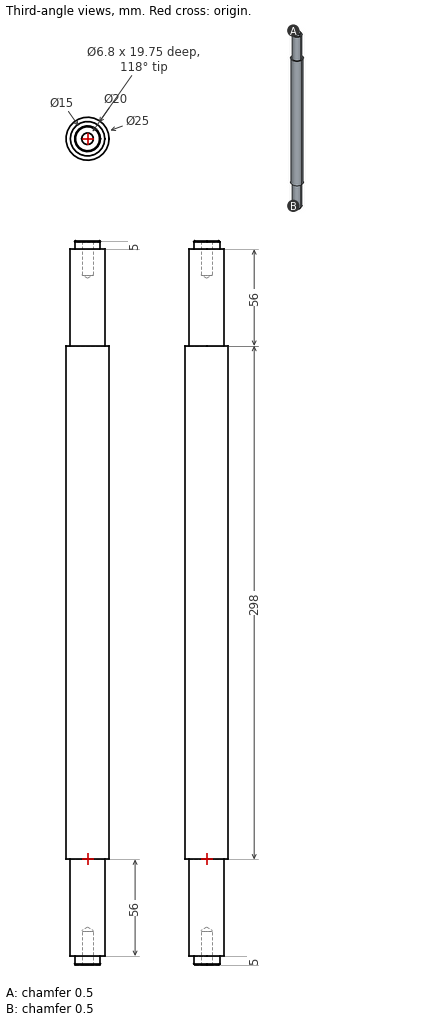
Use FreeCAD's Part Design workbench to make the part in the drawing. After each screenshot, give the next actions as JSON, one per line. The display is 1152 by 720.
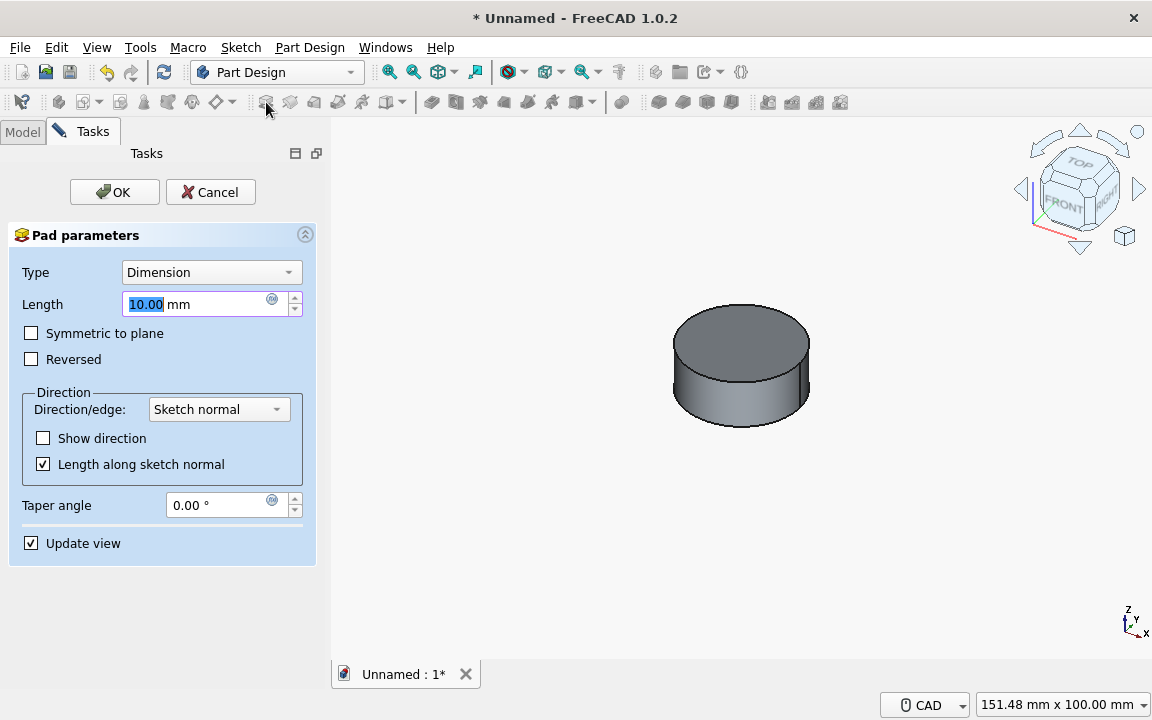
{"action": "type", "text": "298"}
{"action": "key", "text": "Tab"}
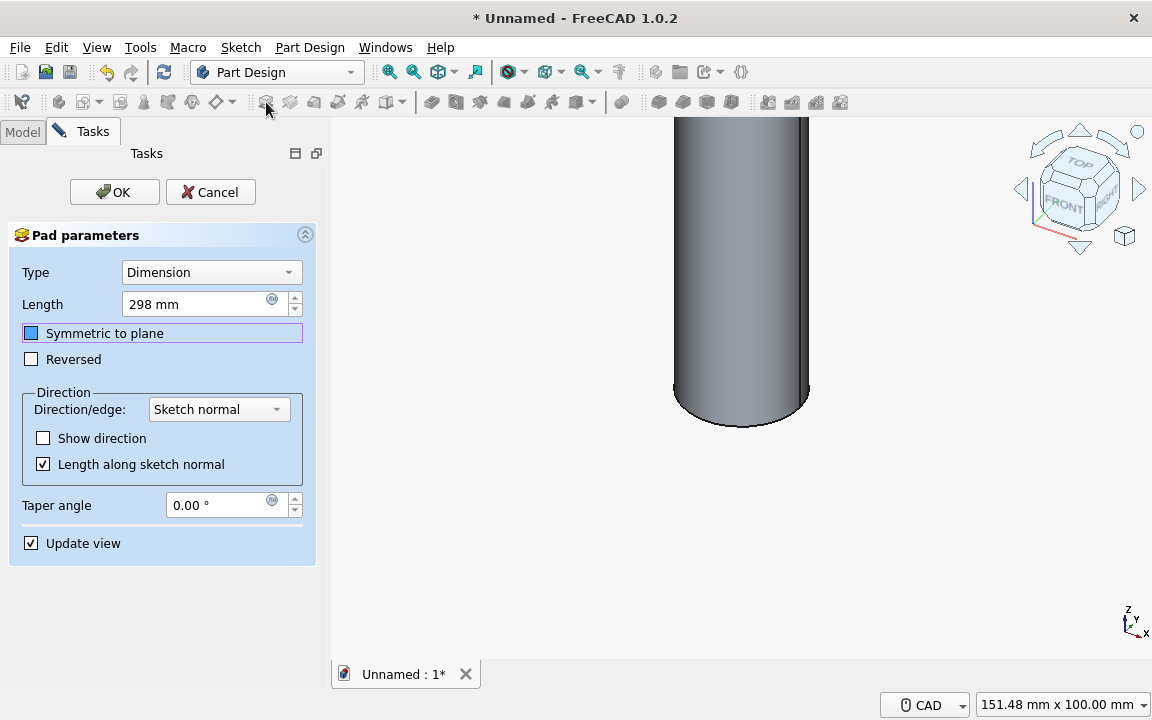
{"action": "left_click", "coordinate": [115, 192]}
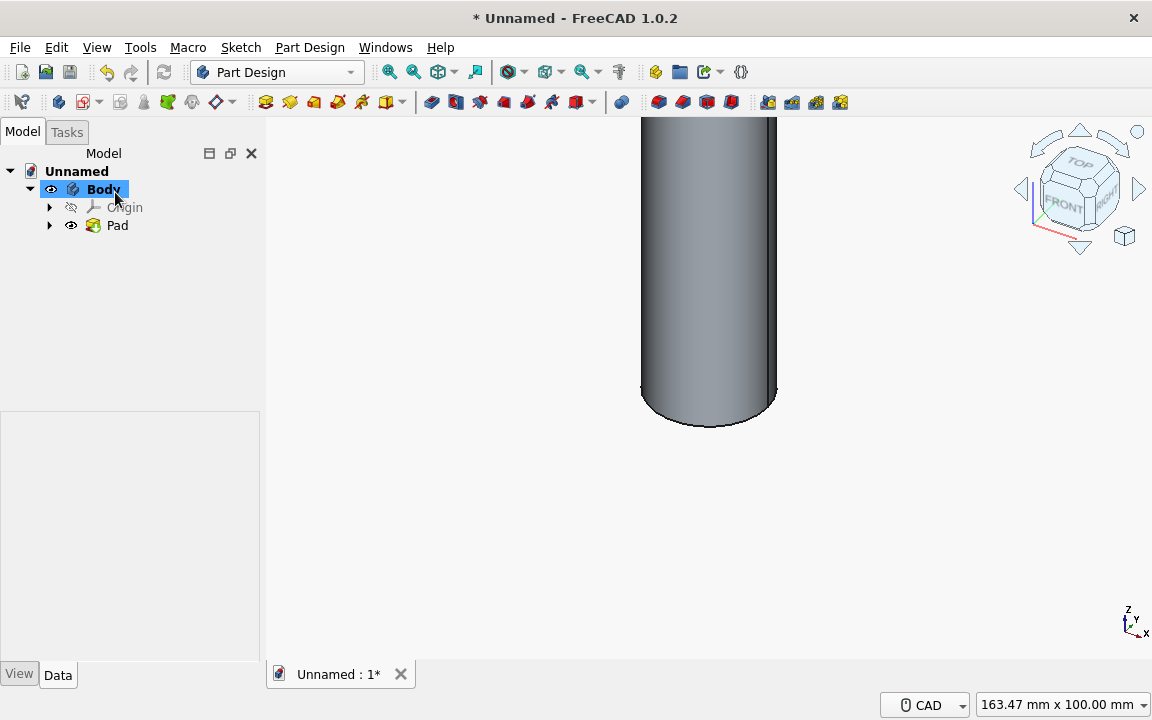
{"action": "left_click", "coordinate": [390, 72]}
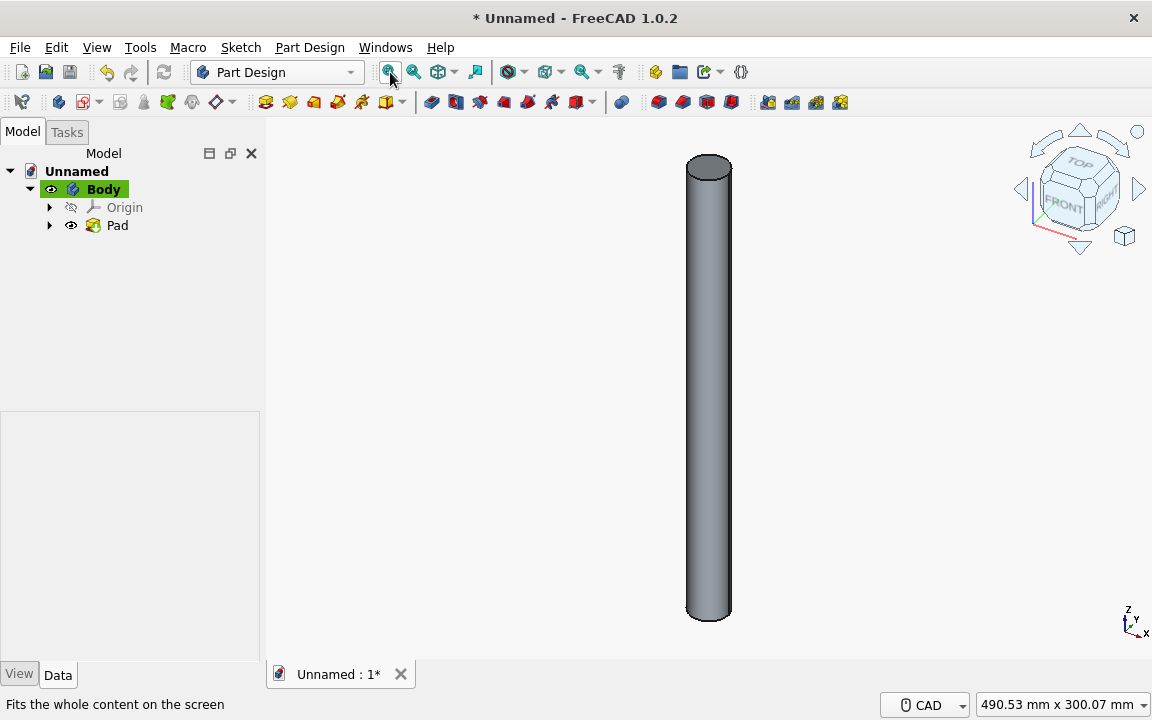
{"action": "key", "text": "5"}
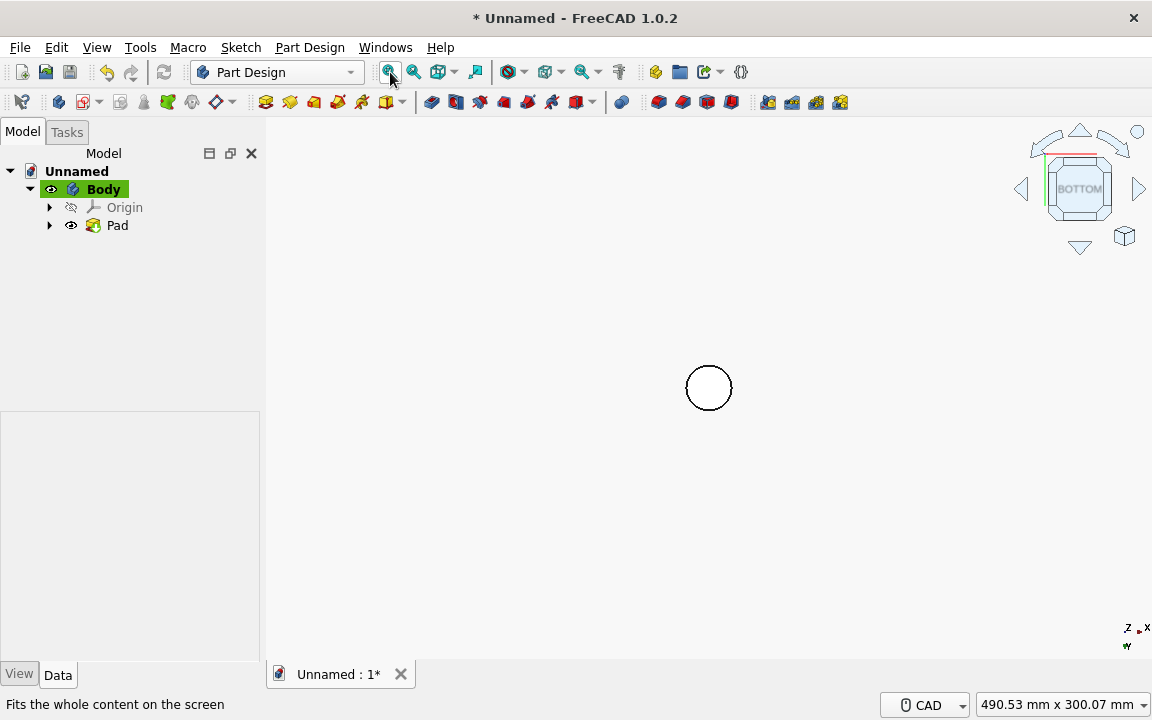
{"action": "left_click", "coordinate": [390, 72]}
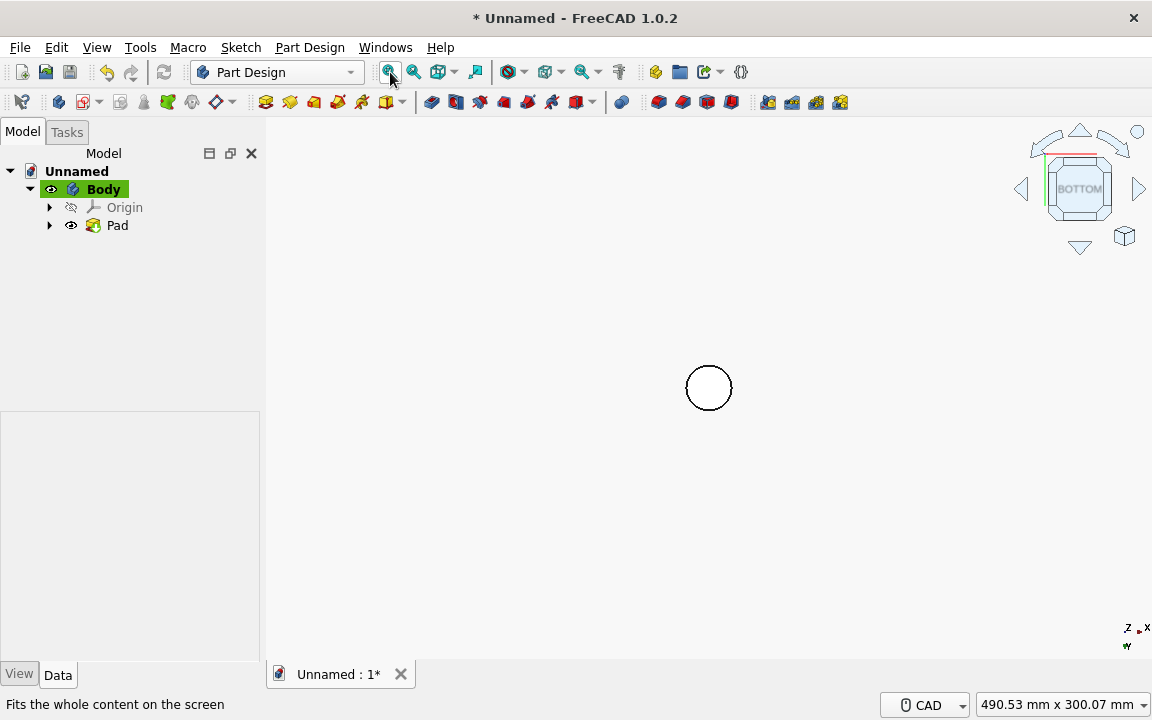
{"action": "left_click", "coordinate": [709, 387]}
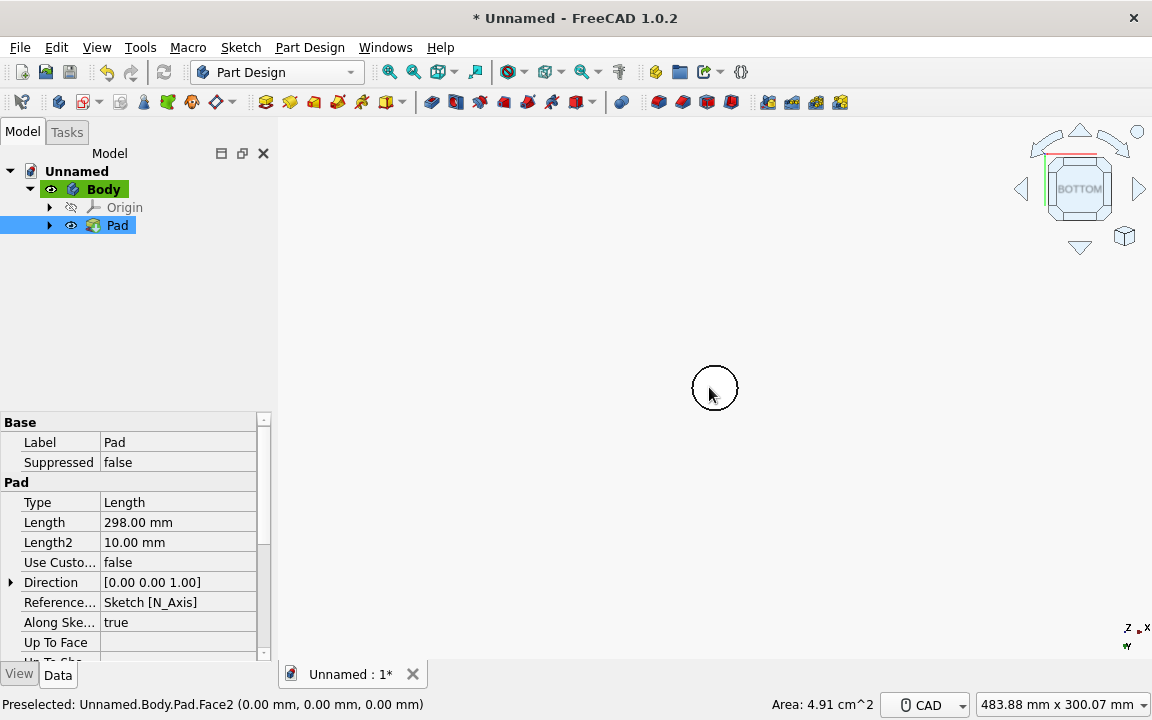
{"action": "left_click", "coordinate": [84, 102]}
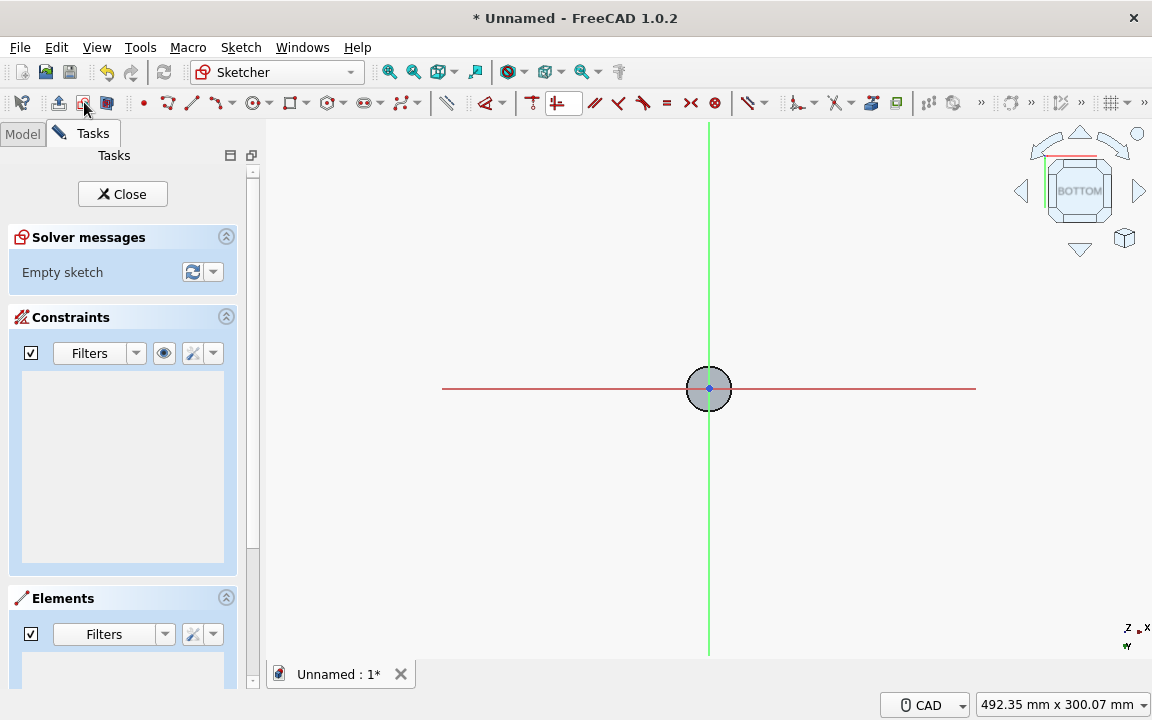
{"action": "scroll", "coordinate": [718, 389], "scroll_direction": "up", "scroll_amount": 11}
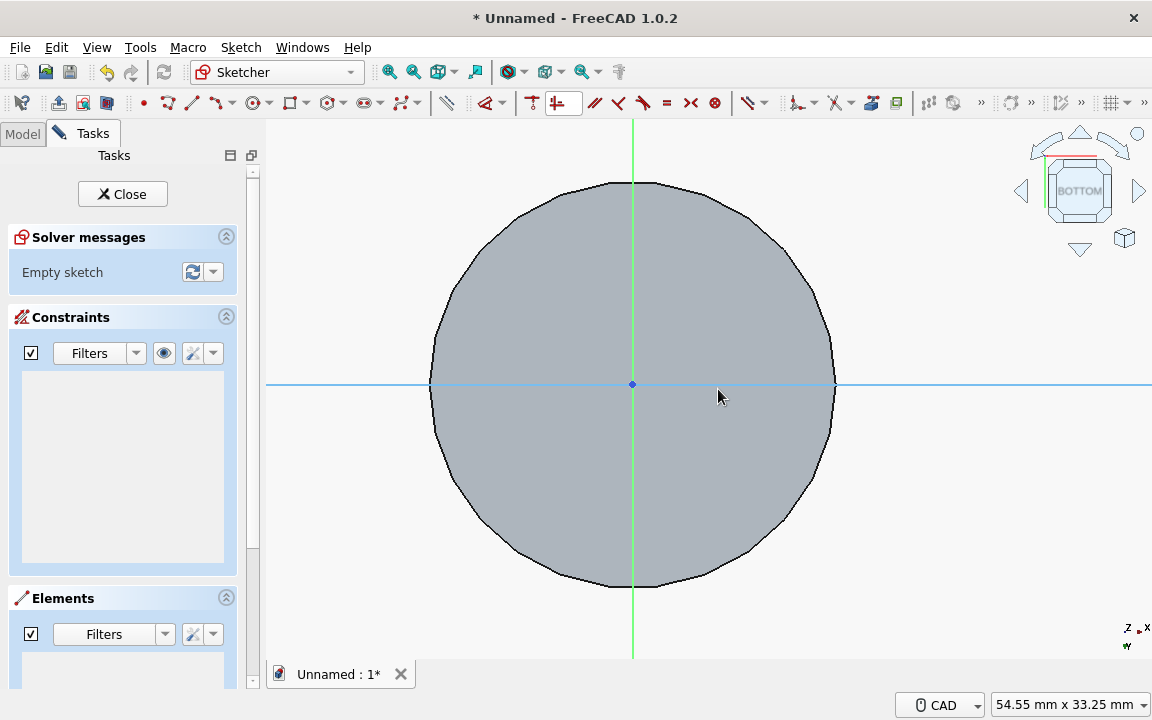
{"action": "left_click", "coordinate": [254, 104]}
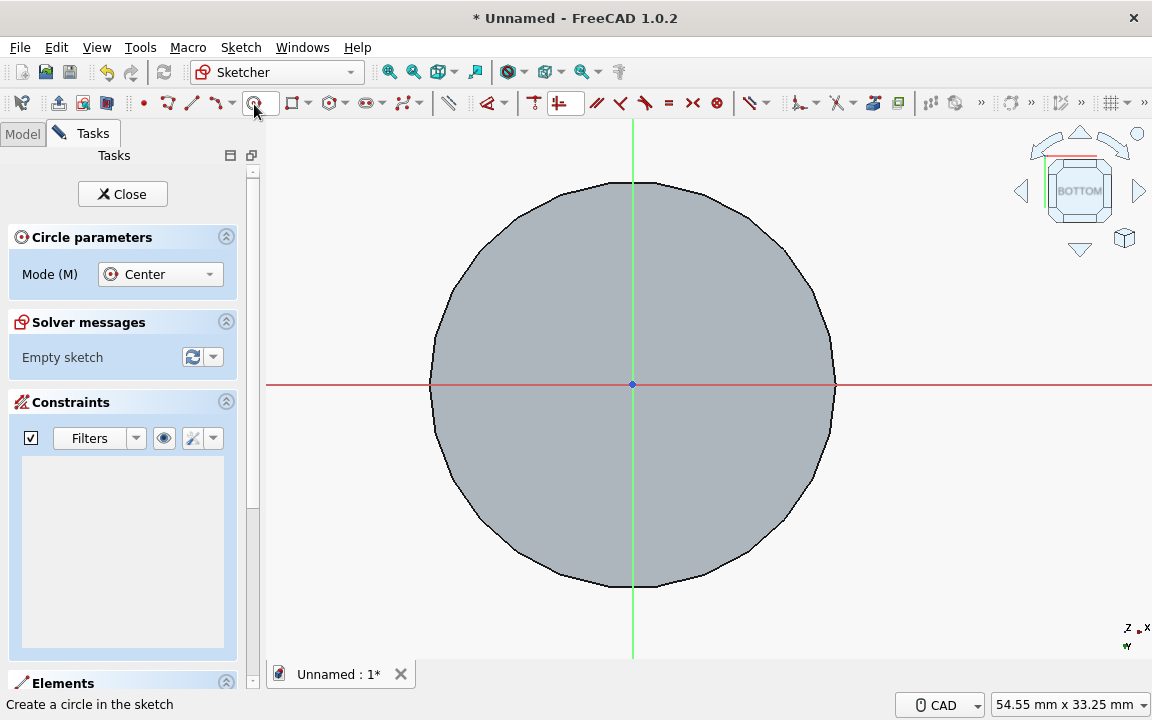
{"action": "left_click", "coordinate": [633, 385]}
{"action": "left_click", "coordinate": [748, 270]}
{"action": "key", "text": "Escape"}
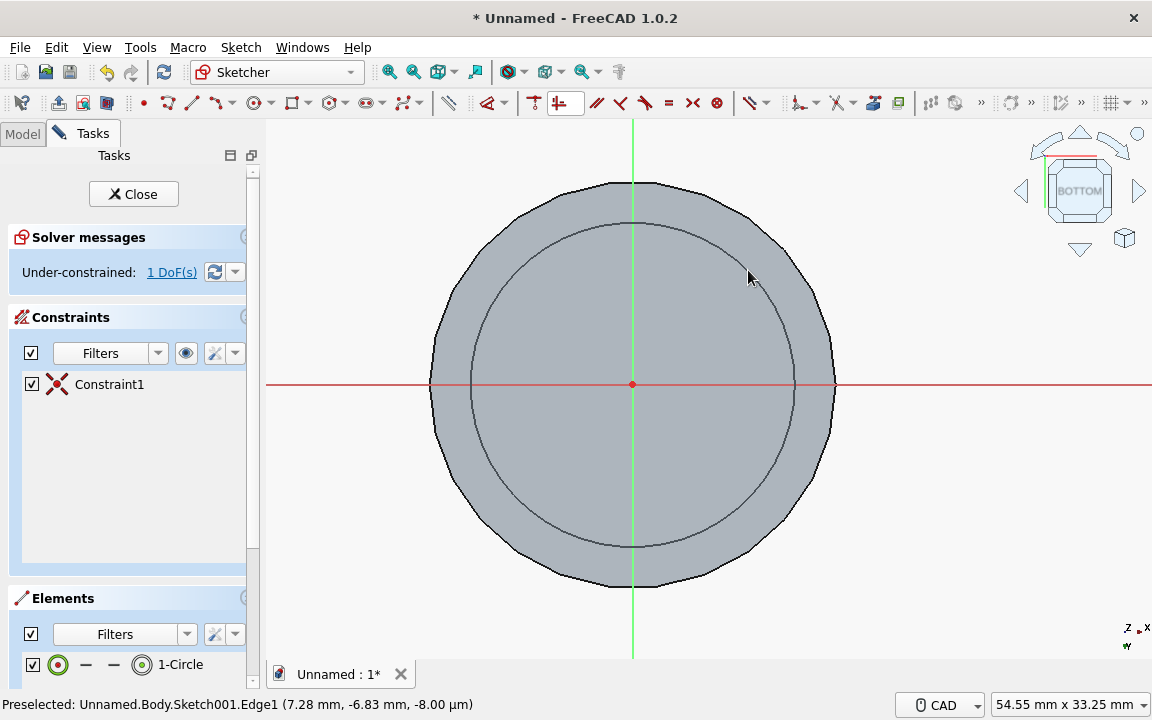
{"action": "left_click", "coordinate": [488, 104]}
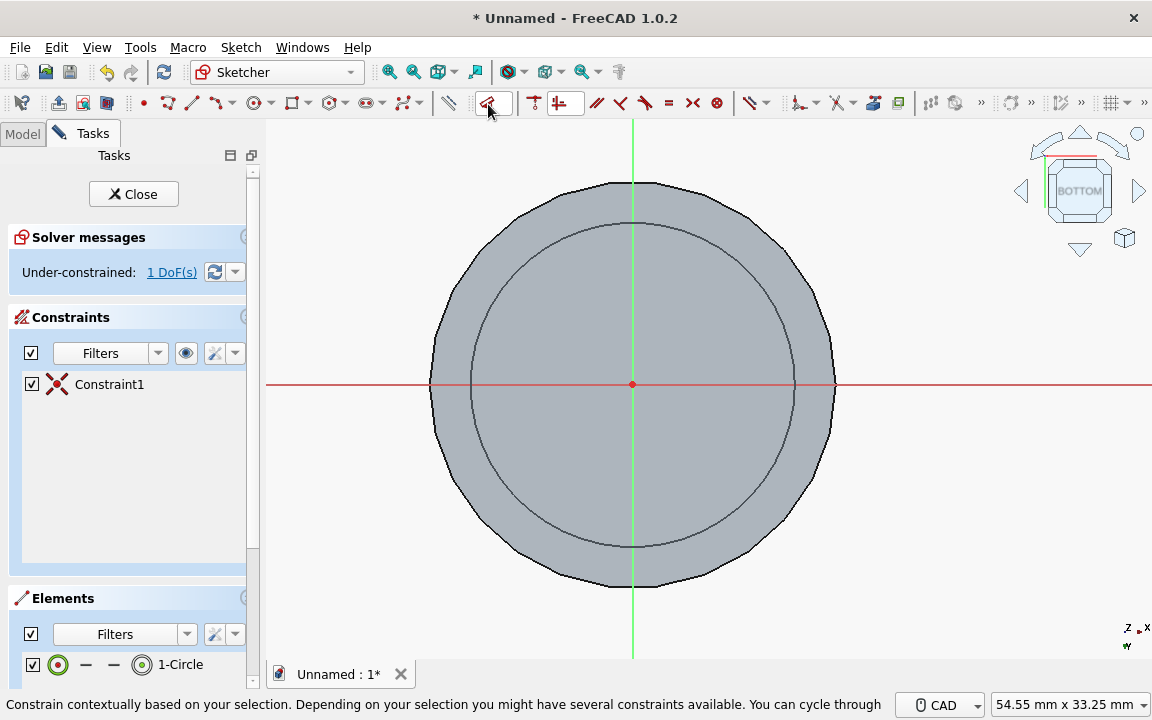
{"action": "left_click", "coordinate": [747, 270]}
{"action": "left_click", "coordinate": [770, 247]}